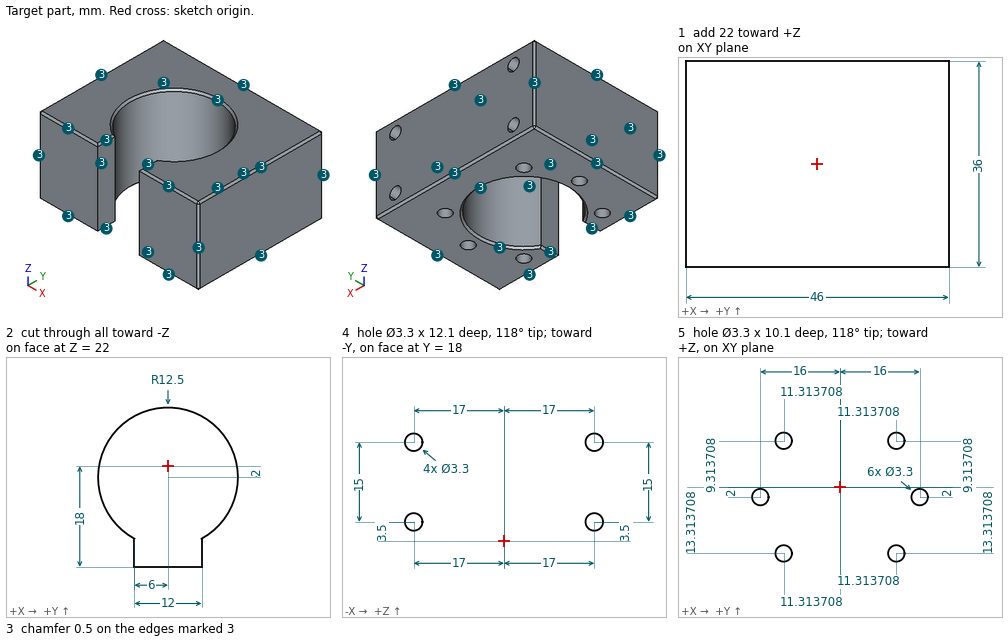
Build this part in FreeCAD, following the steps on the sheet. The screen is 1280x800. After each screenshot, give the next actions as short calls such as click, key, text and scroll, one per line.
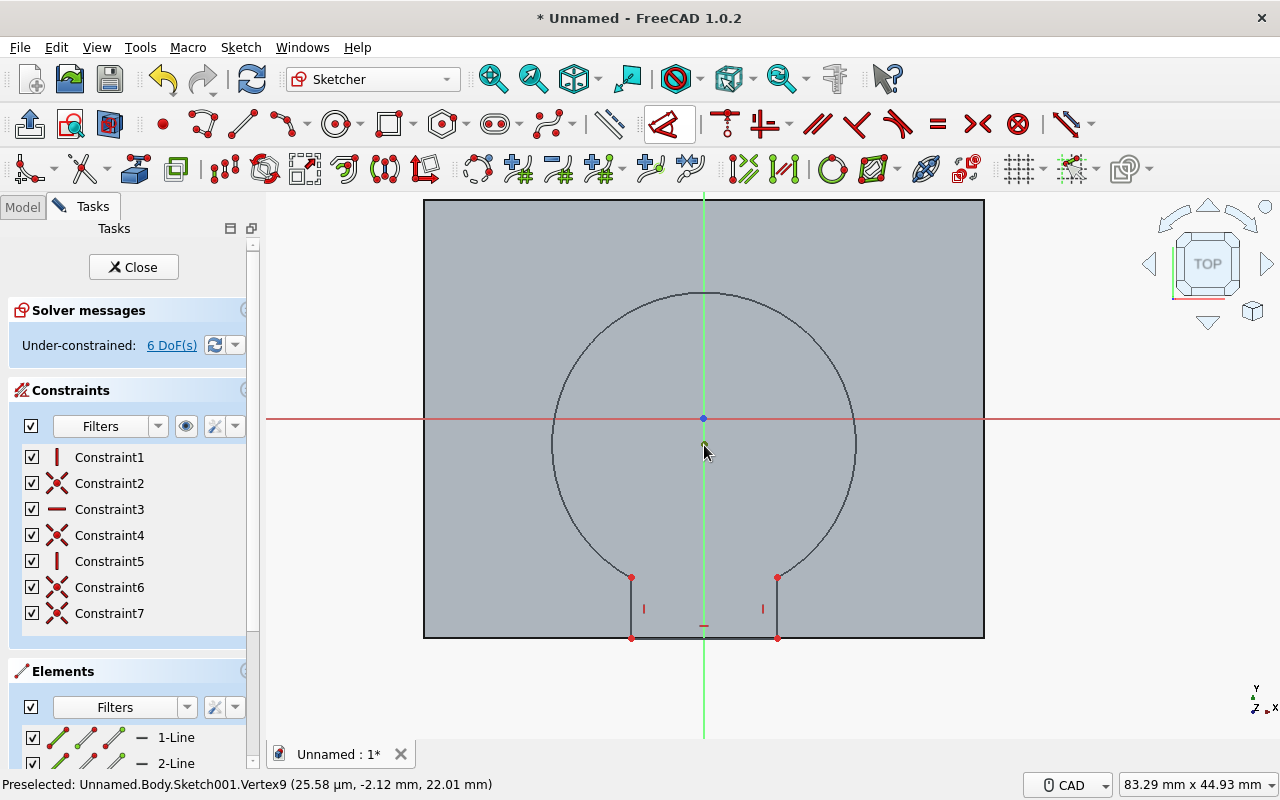
click(704, 676)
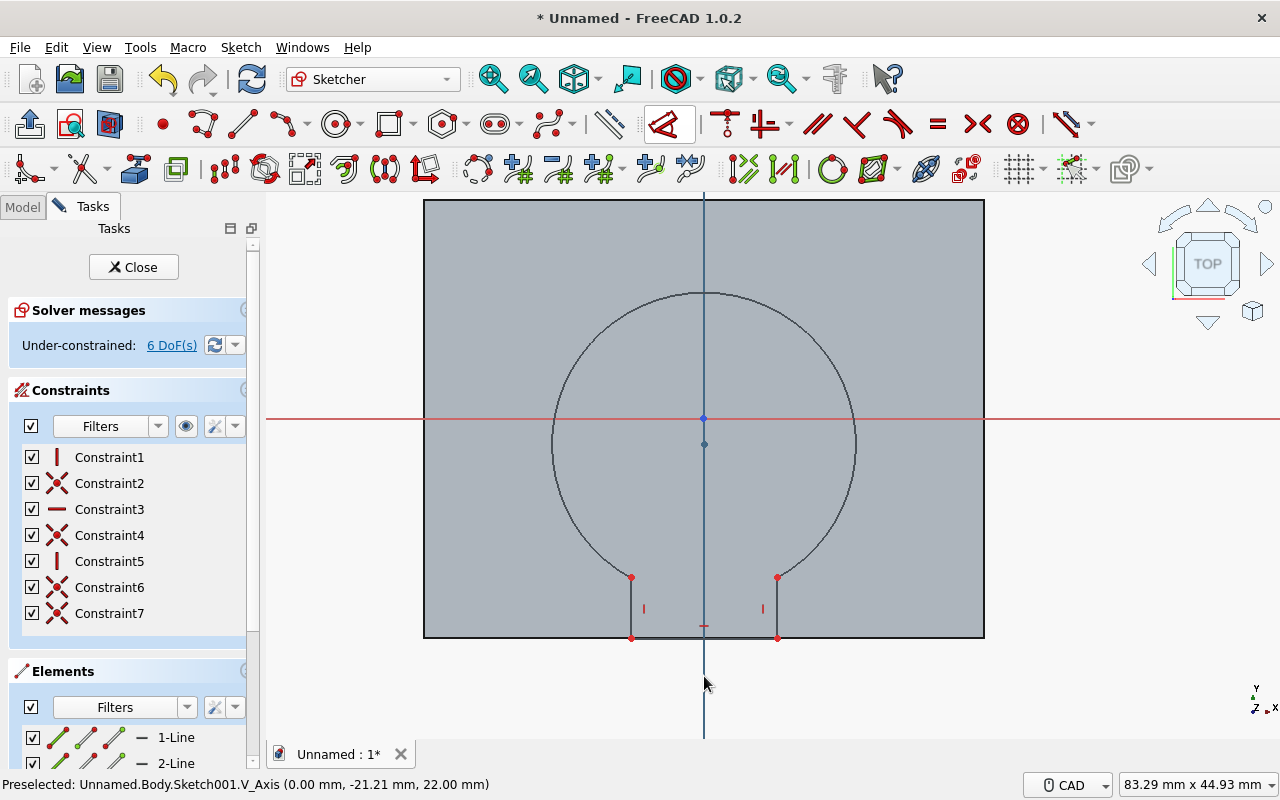
click(726, 124)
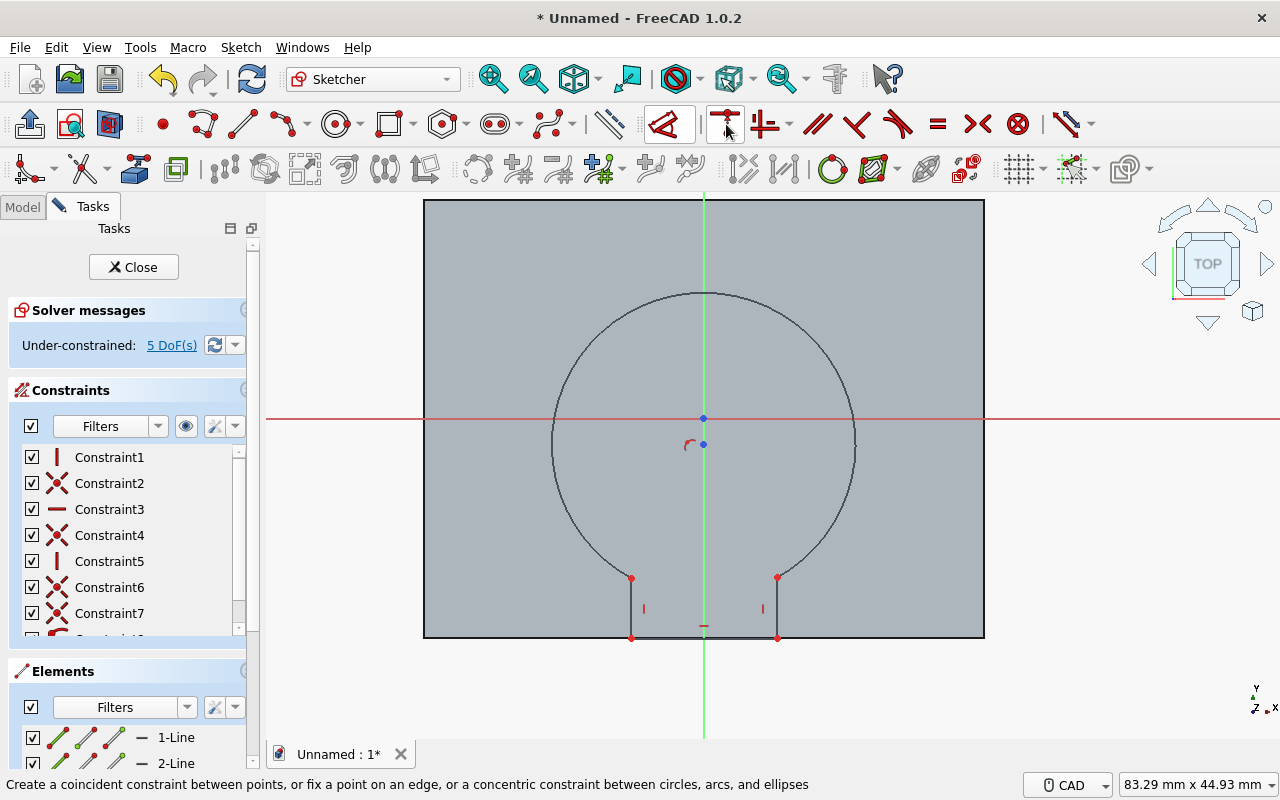
click(664, 124)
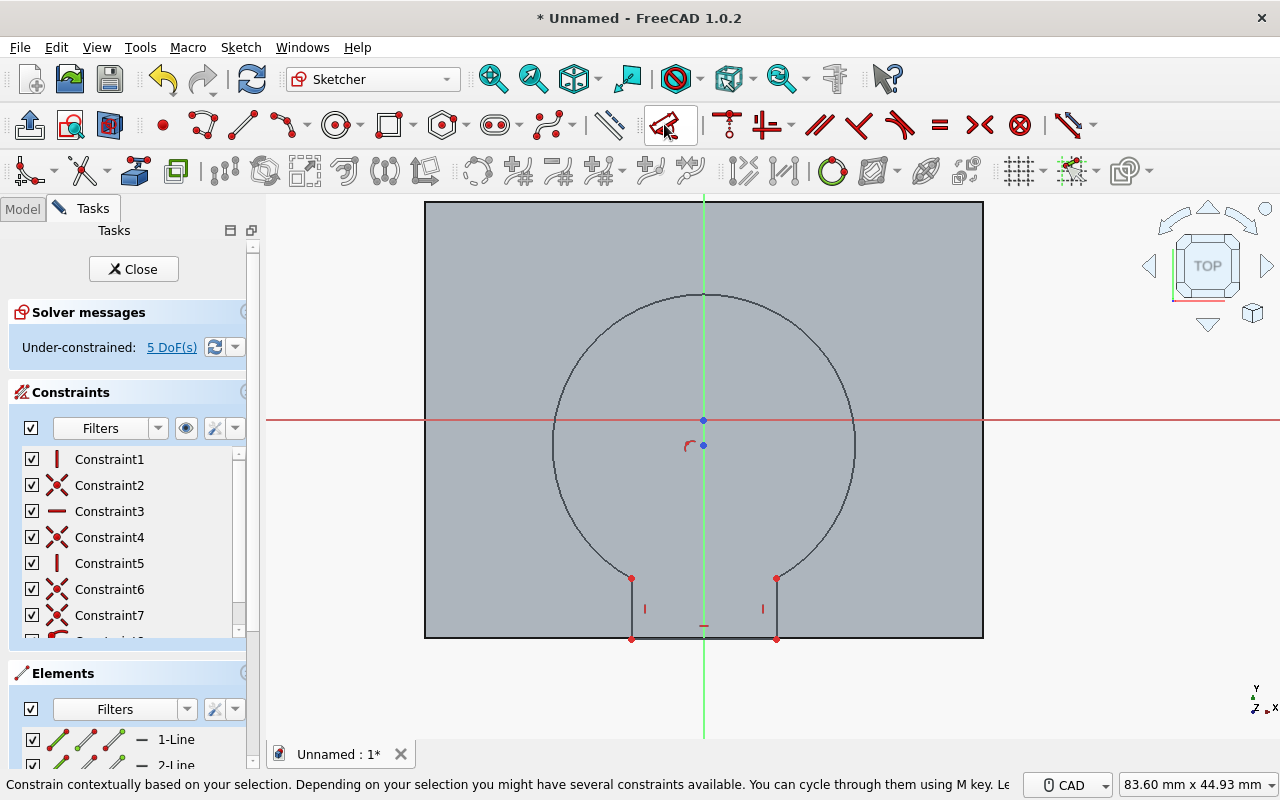
click(835, 371)
click(863, 355)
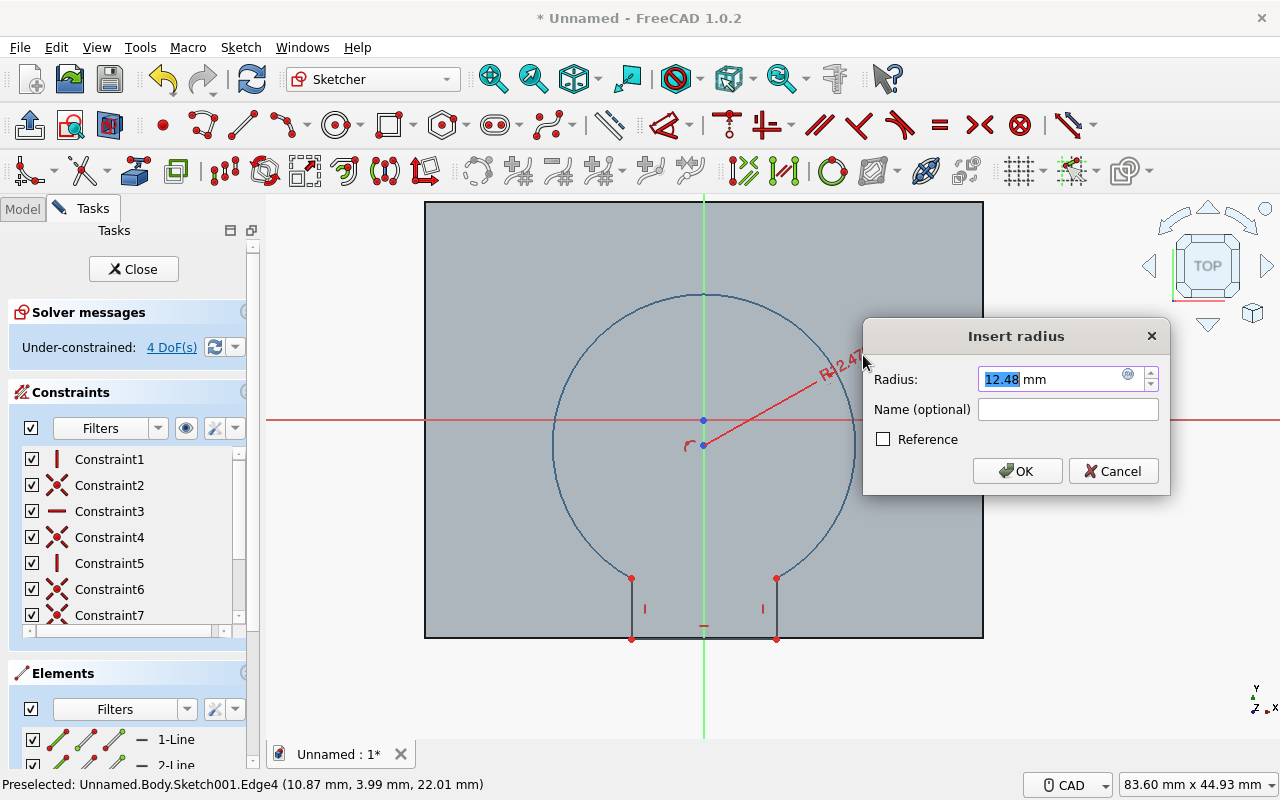
text(12.5)
key(Return)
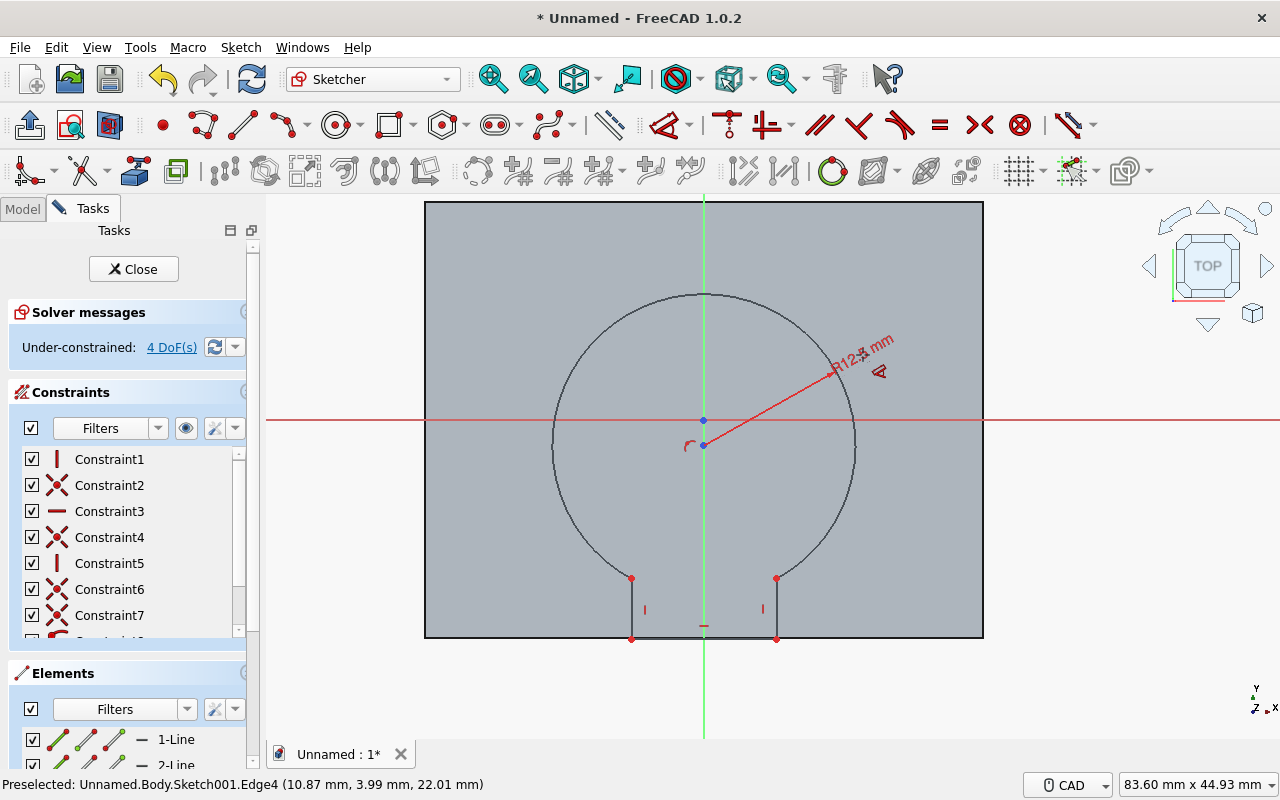
click(675, 639)
click(671, 673)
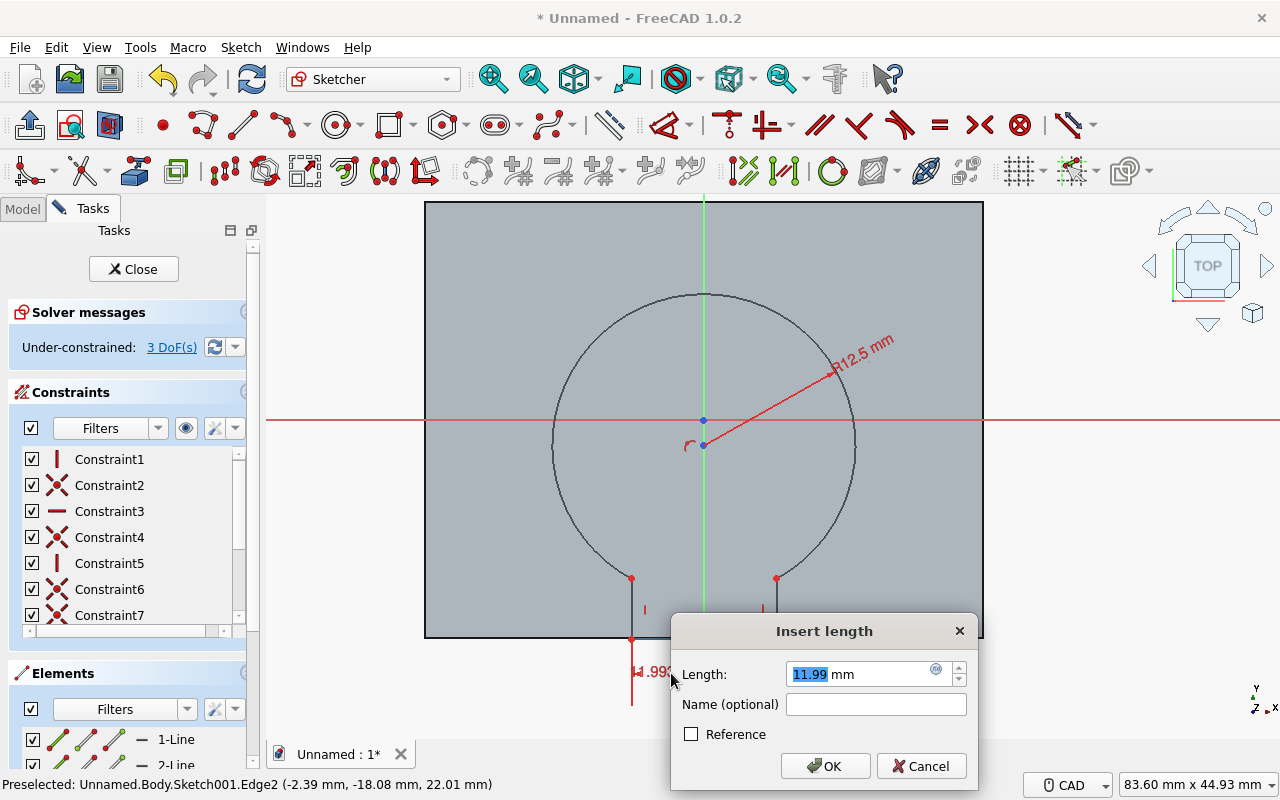
text(12)
key(Return)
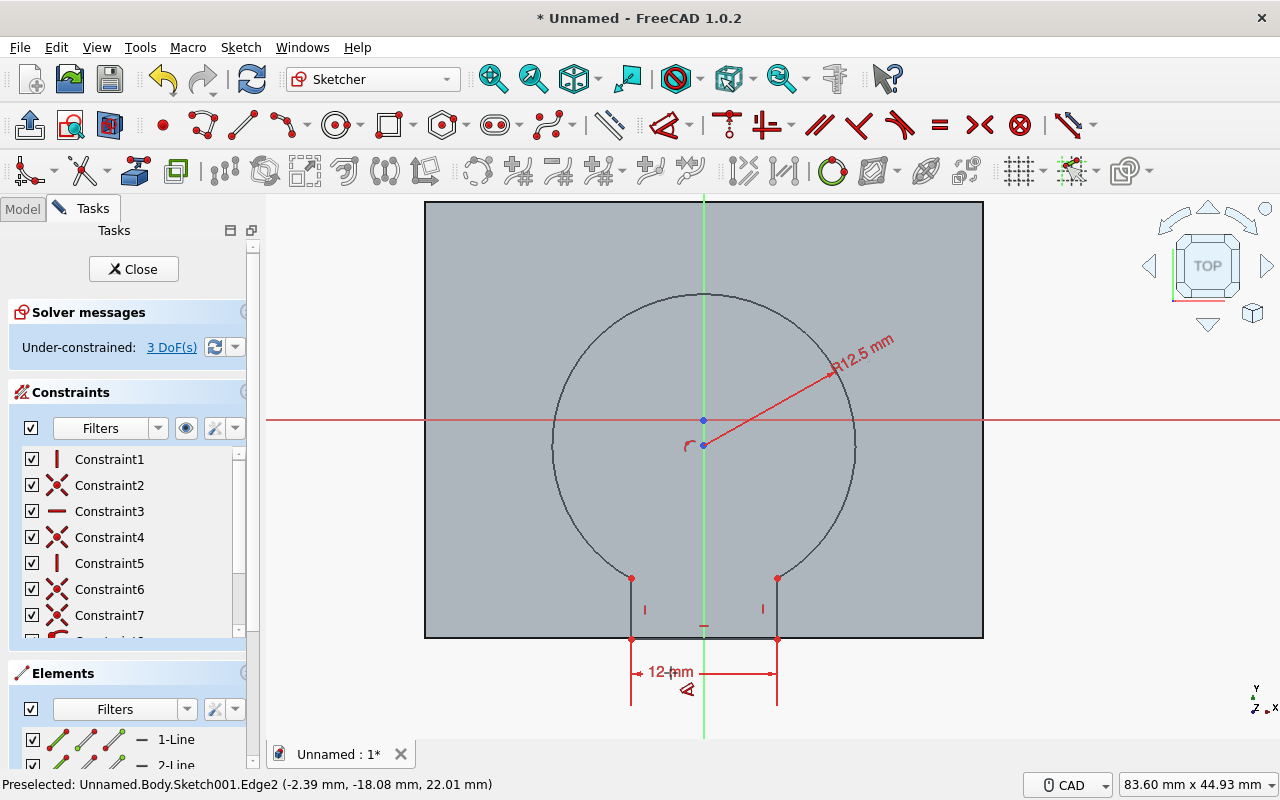
click(631, 579)
click(668, 613)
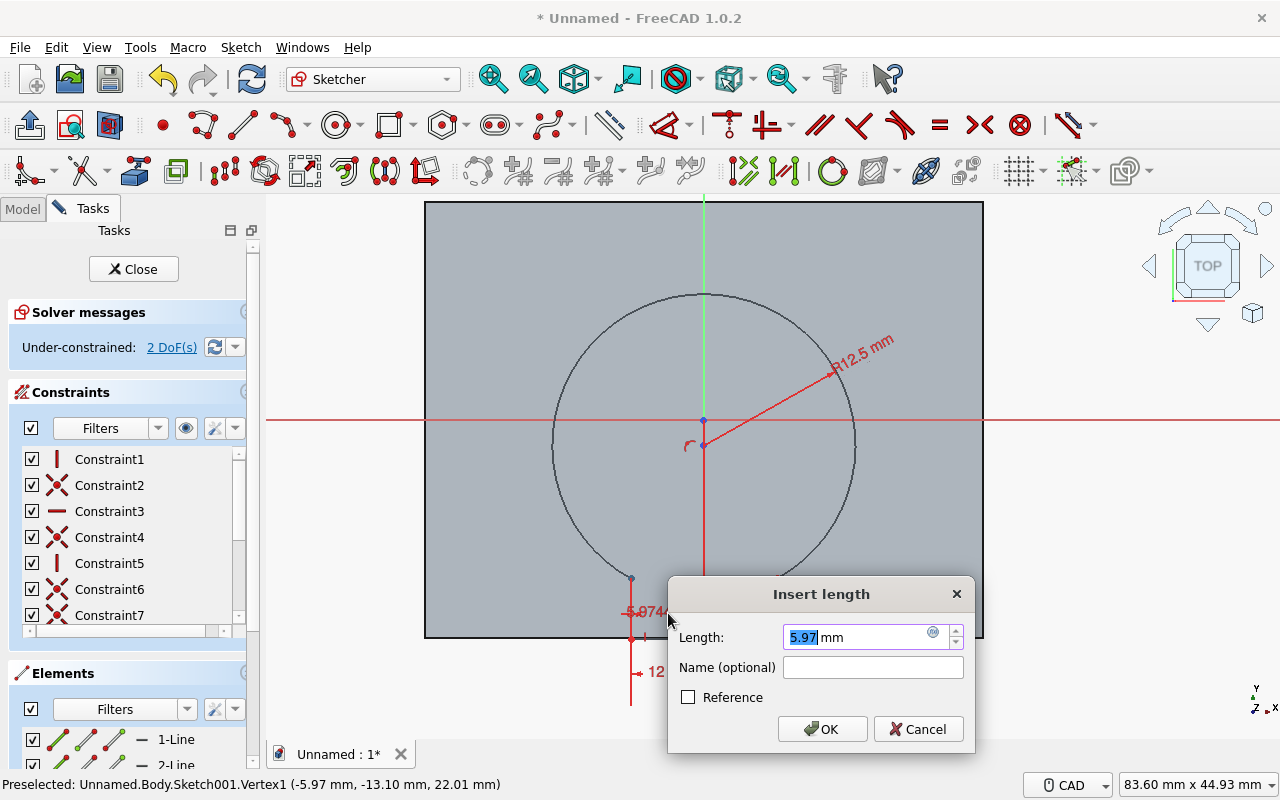
text(6)
key(Return)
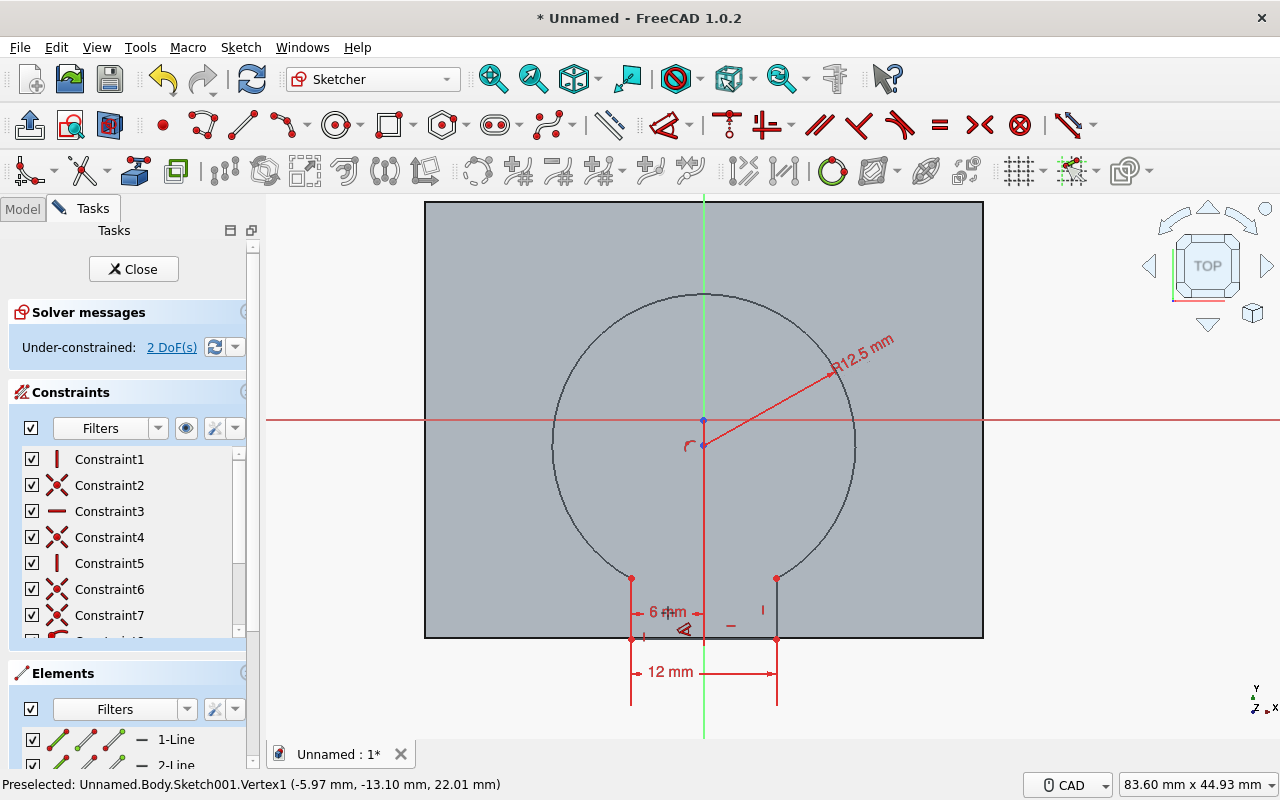
scroll(704, 446, up, 3)